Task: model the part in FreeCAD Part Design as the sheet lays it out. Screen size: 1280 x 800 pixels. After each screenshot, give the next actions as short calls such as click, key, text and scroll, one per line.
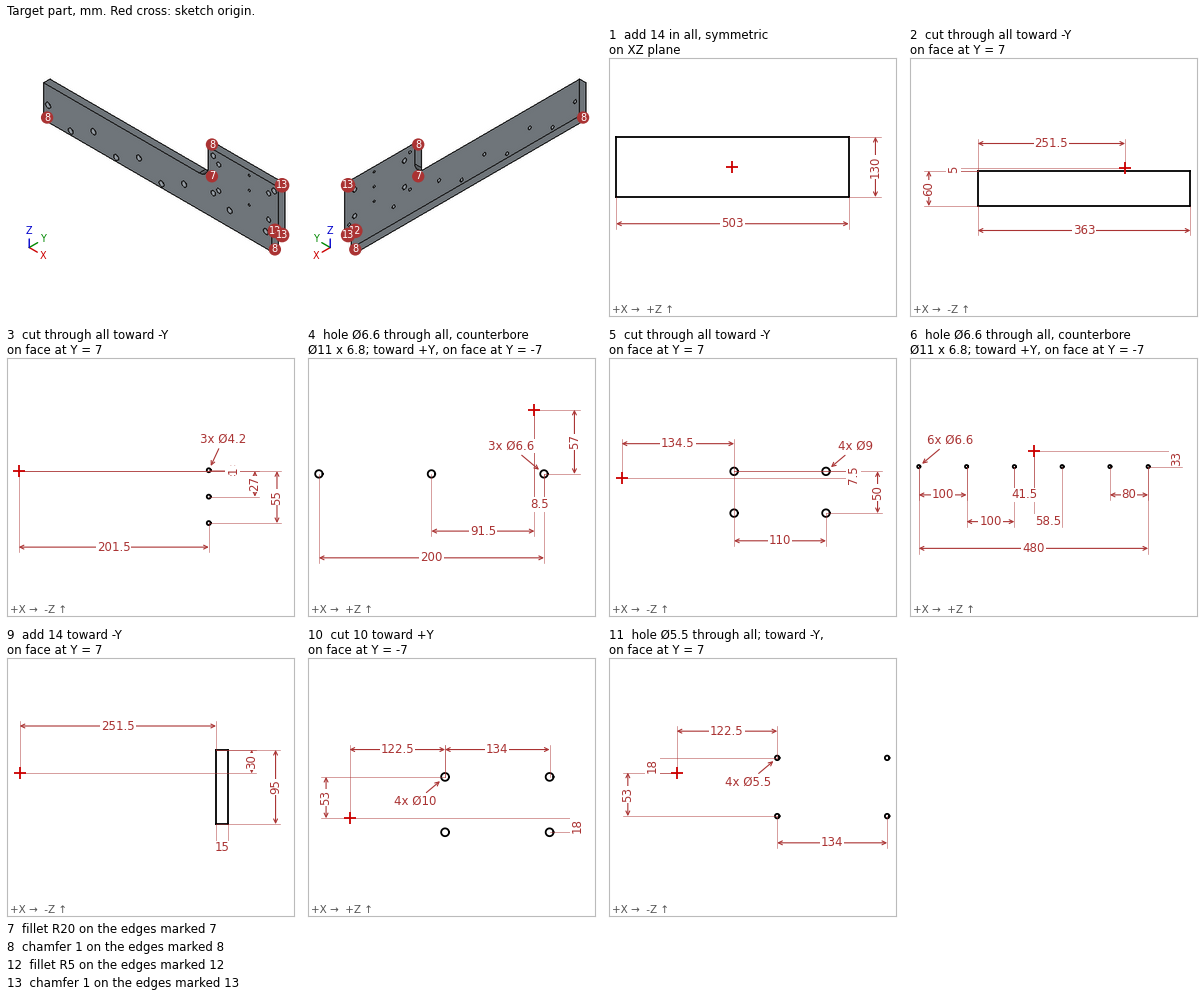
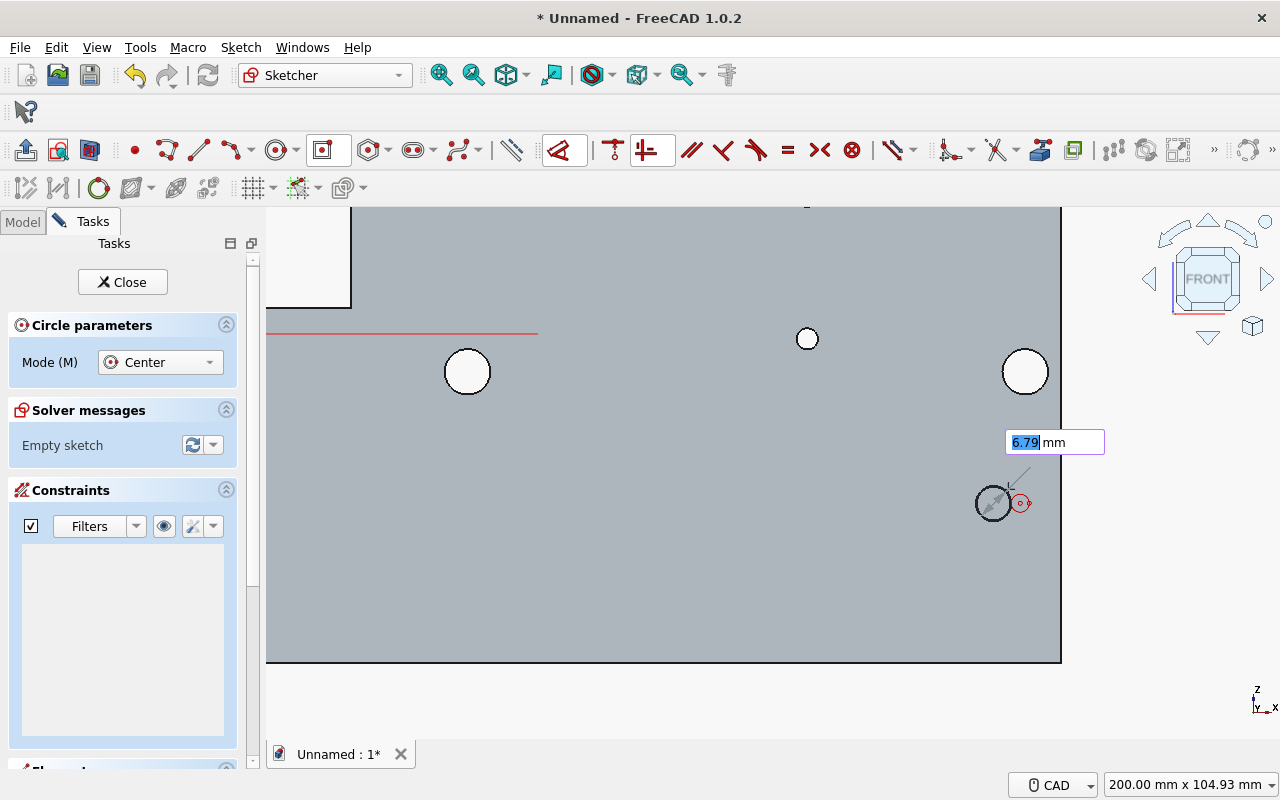
click(1007, 489)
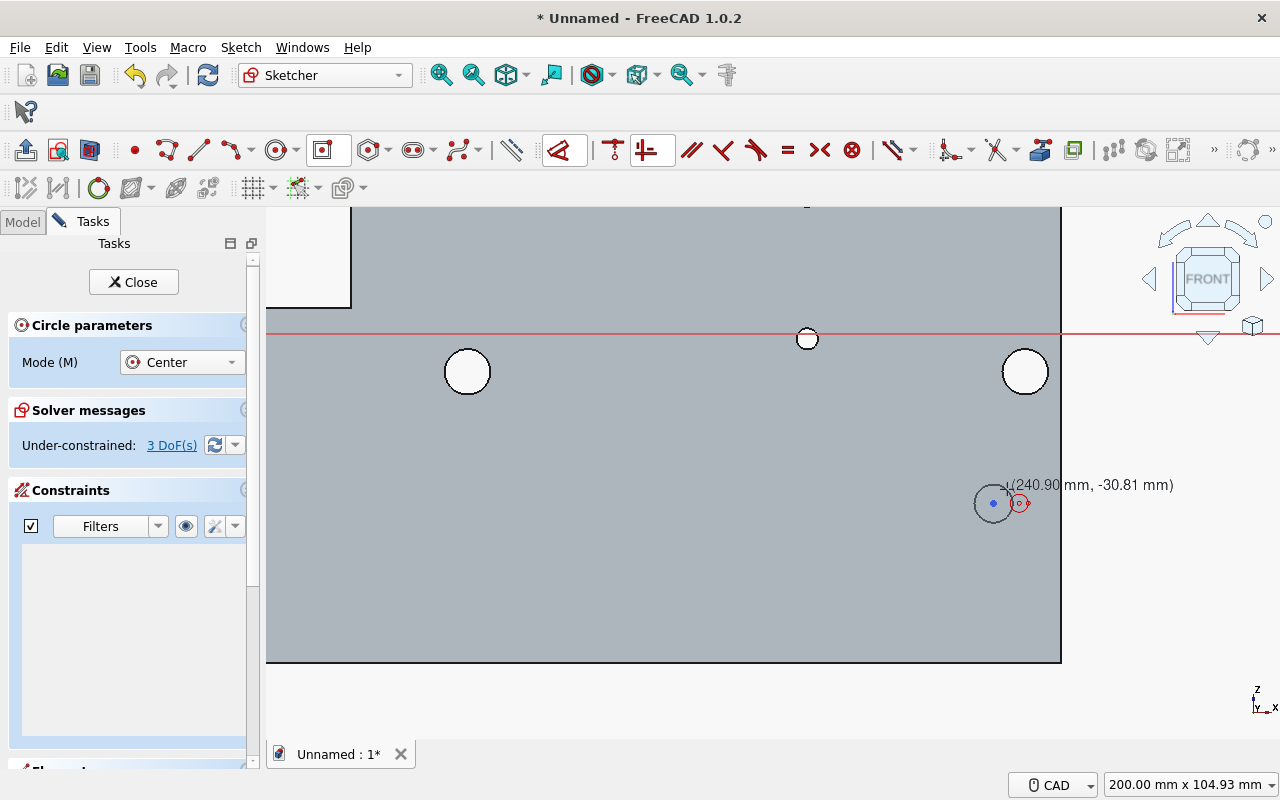
scroll(1008, 488, down, 7)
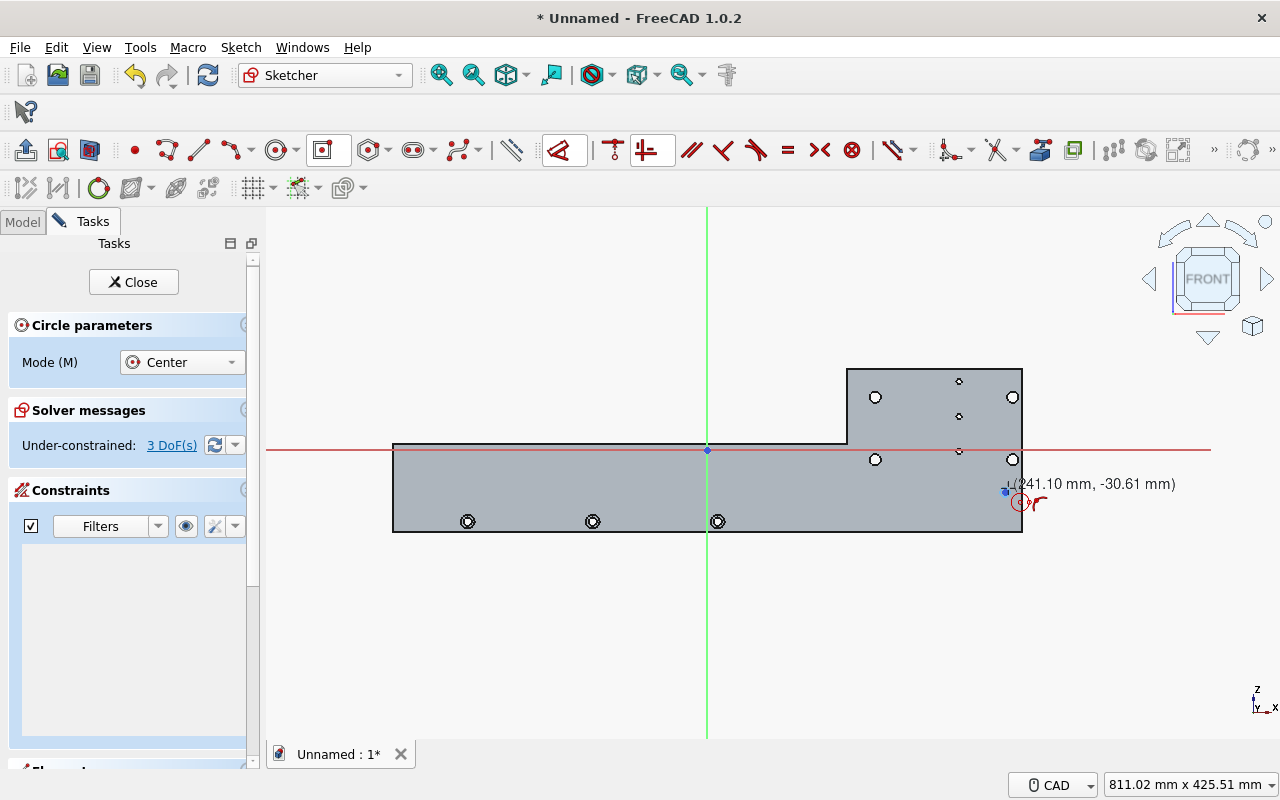
scroll(405, 492, up, 9)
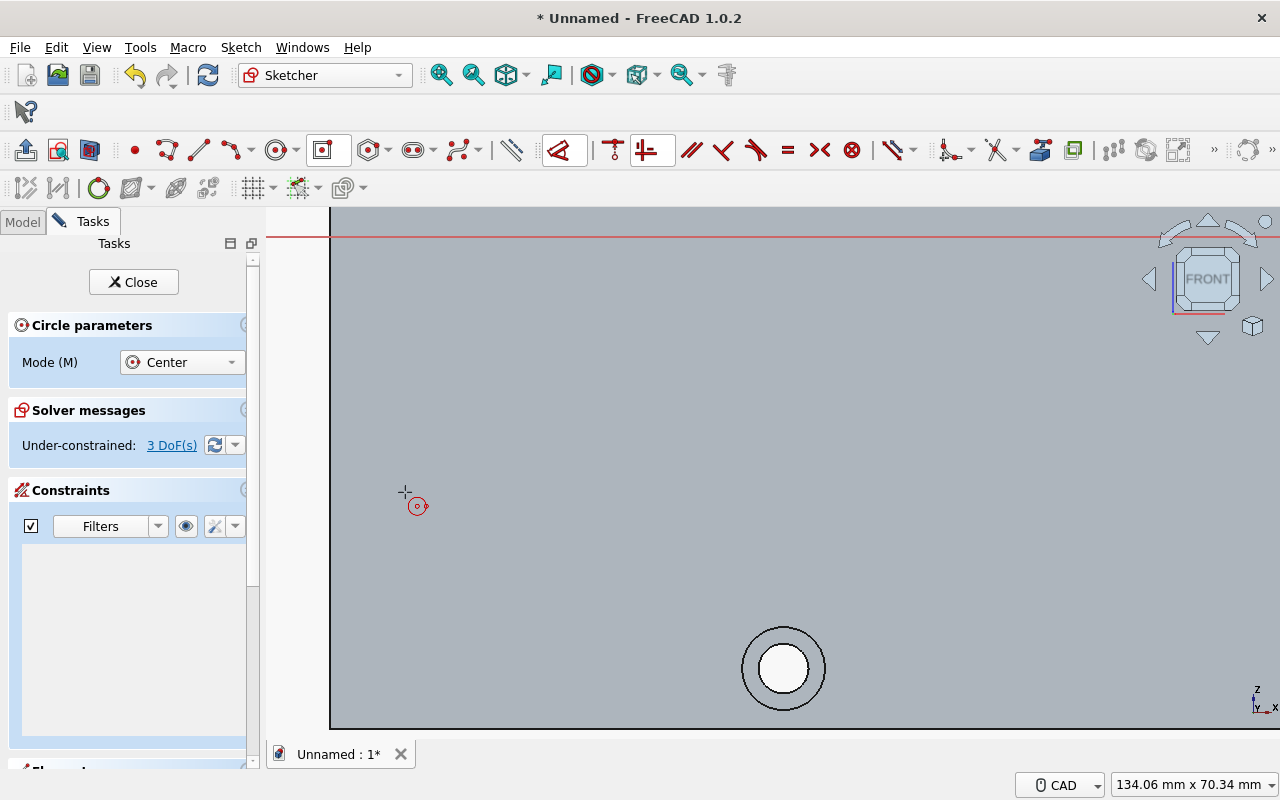
scroll(404, 492, down, 9)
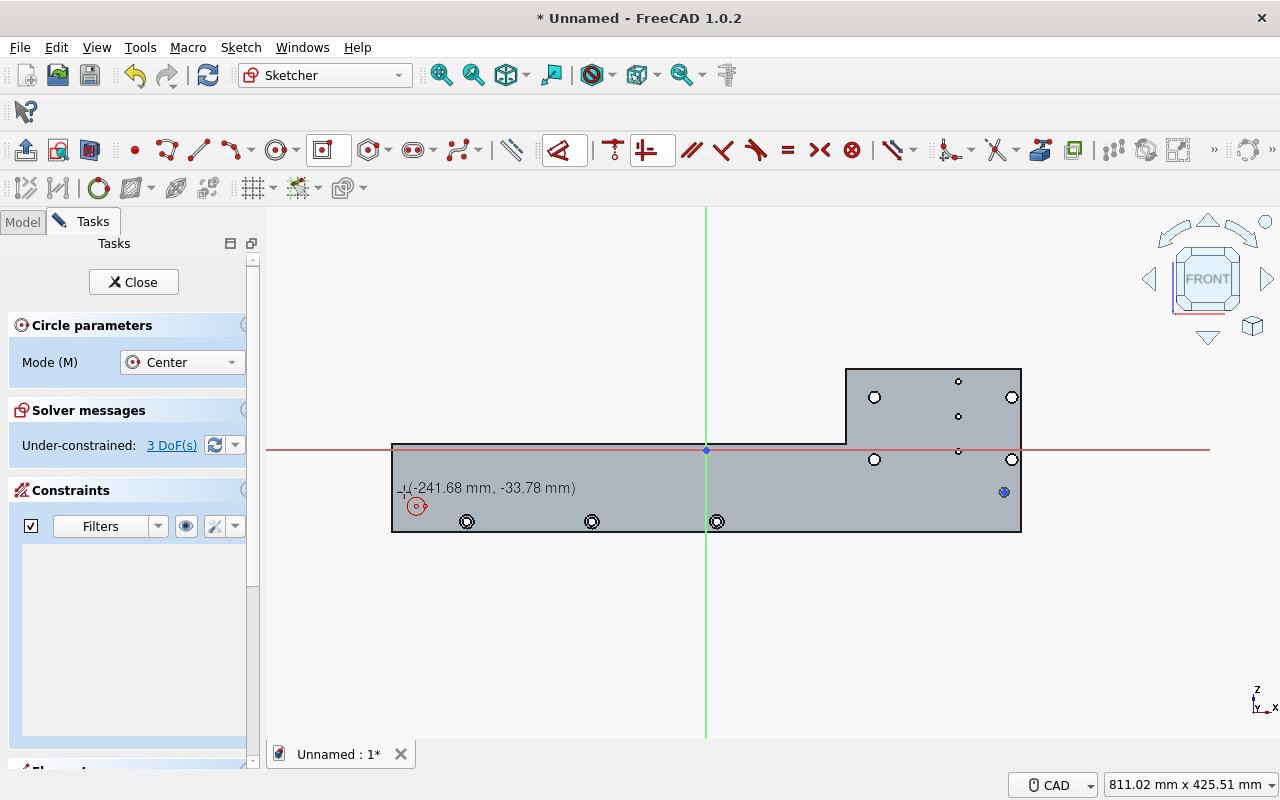
click(404, 492)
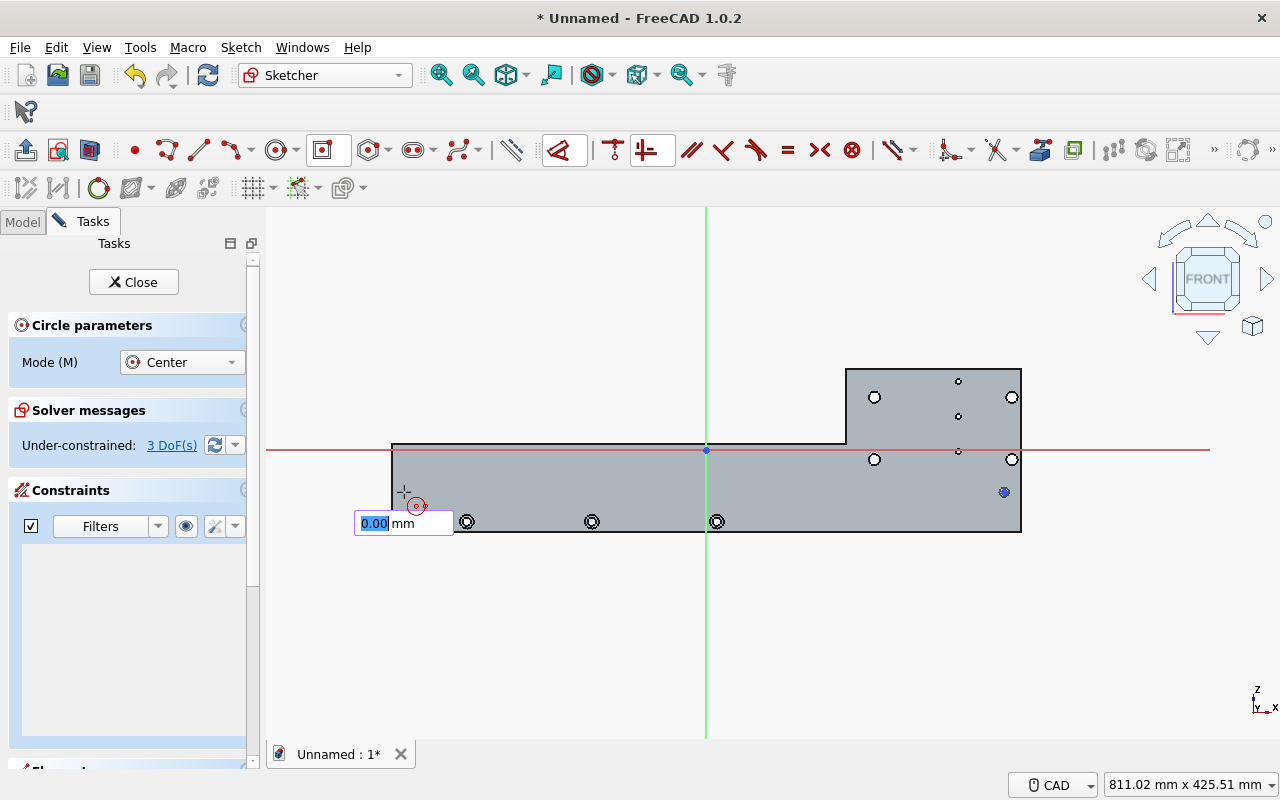
scroll(407, 489, up, 7)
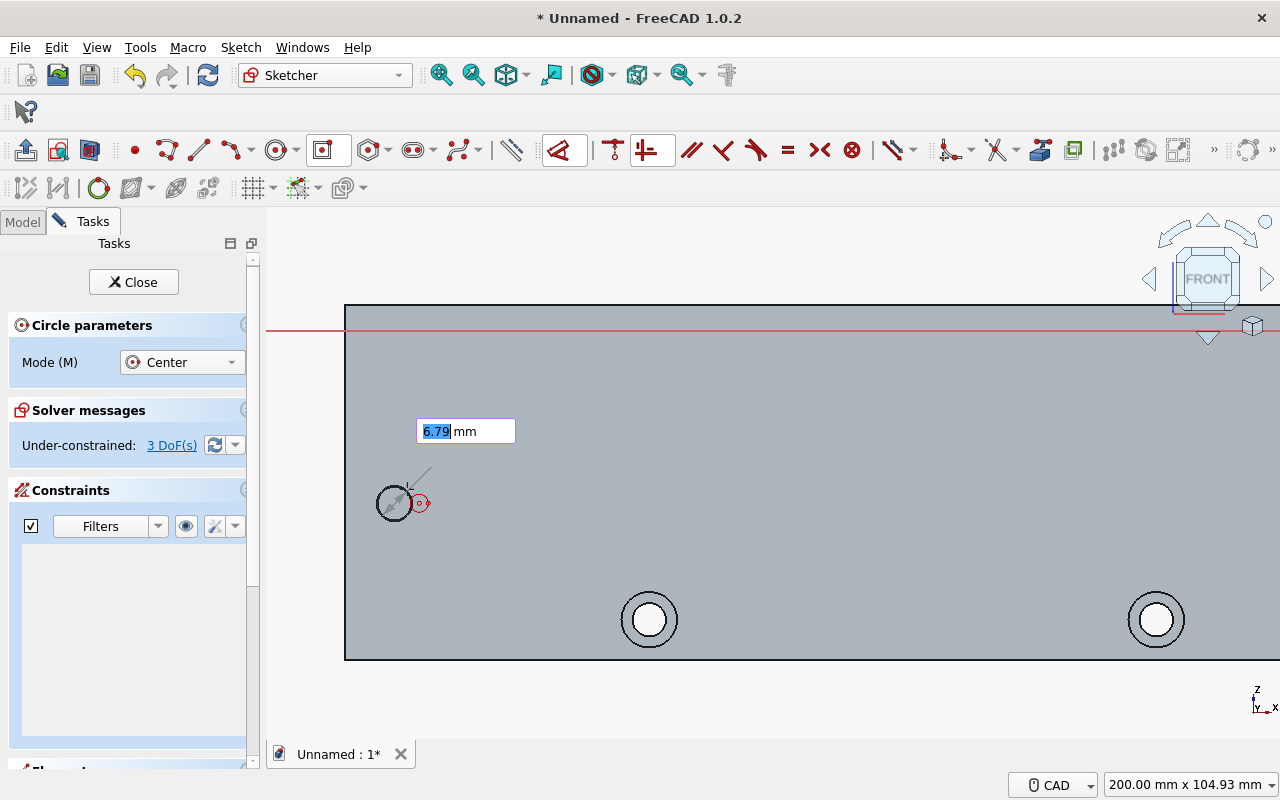
click(408, 486)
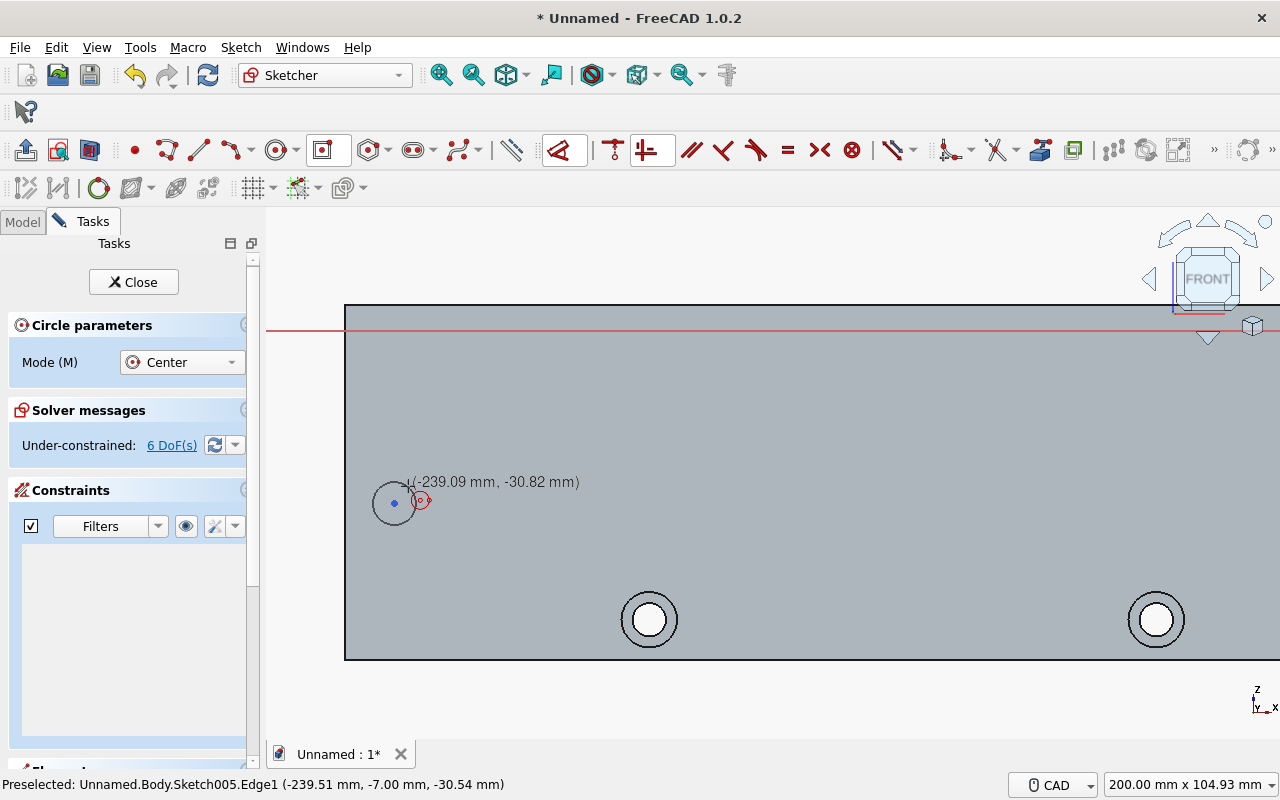
scroll(903, 498, up, 2)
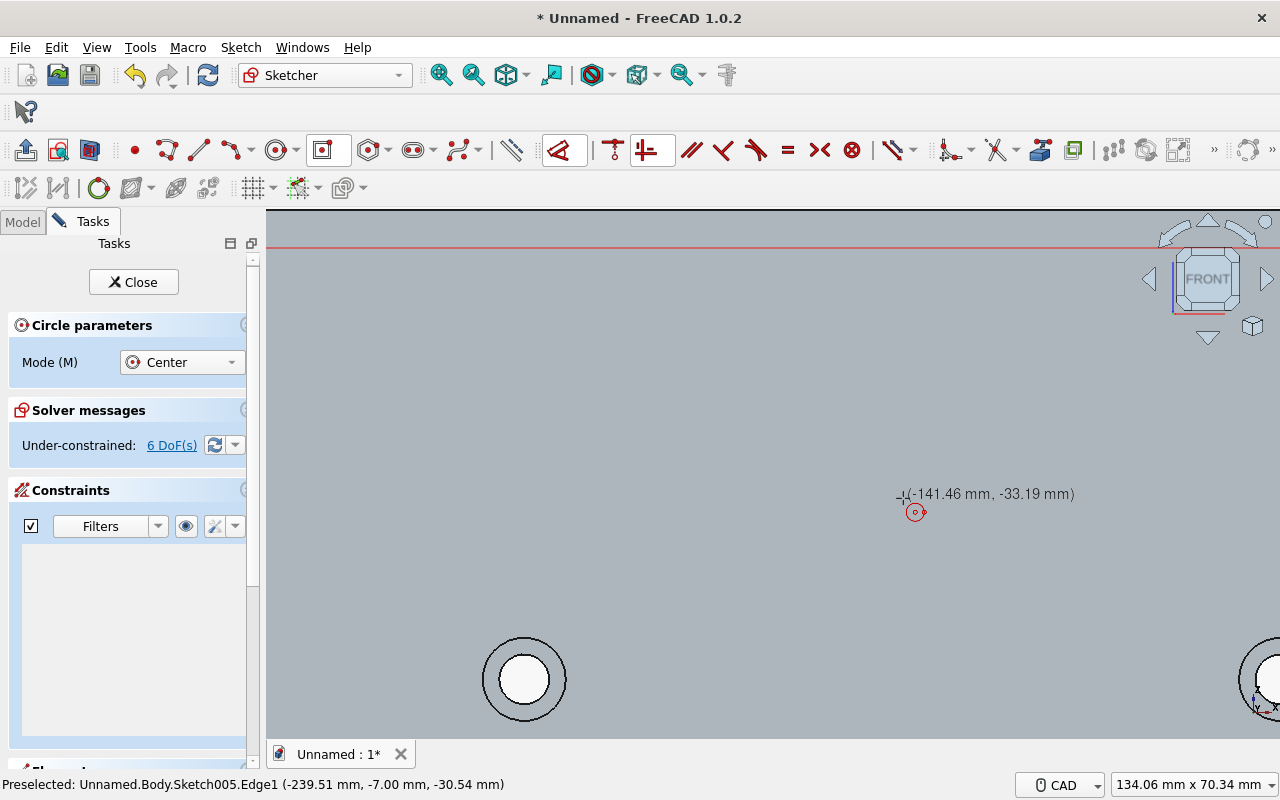
scroll(456, 490, down, 9)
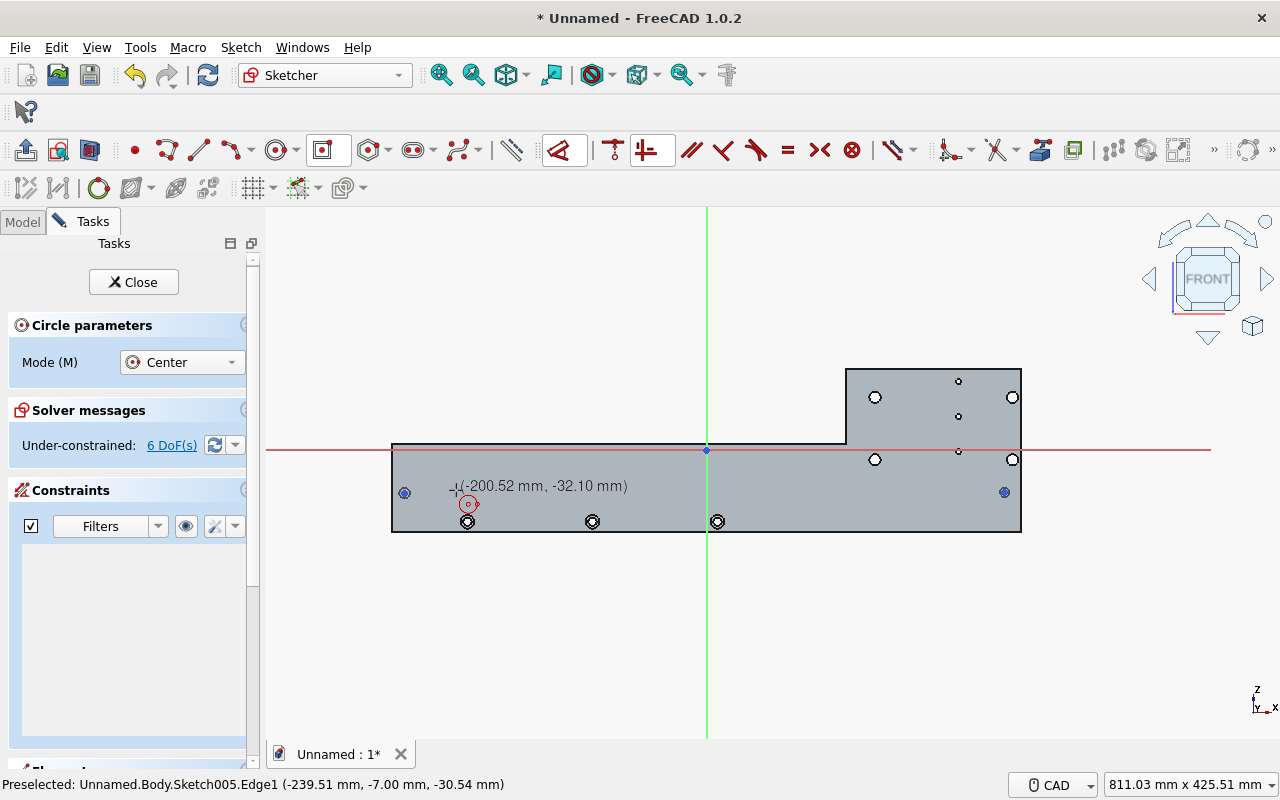
click(530, 492)